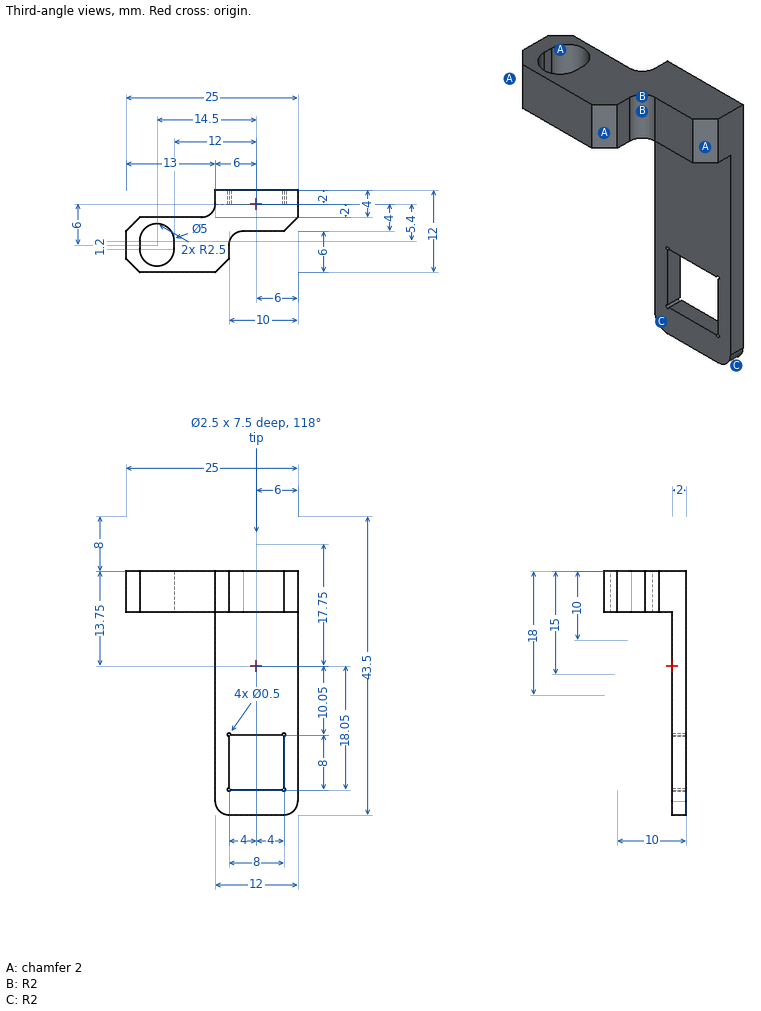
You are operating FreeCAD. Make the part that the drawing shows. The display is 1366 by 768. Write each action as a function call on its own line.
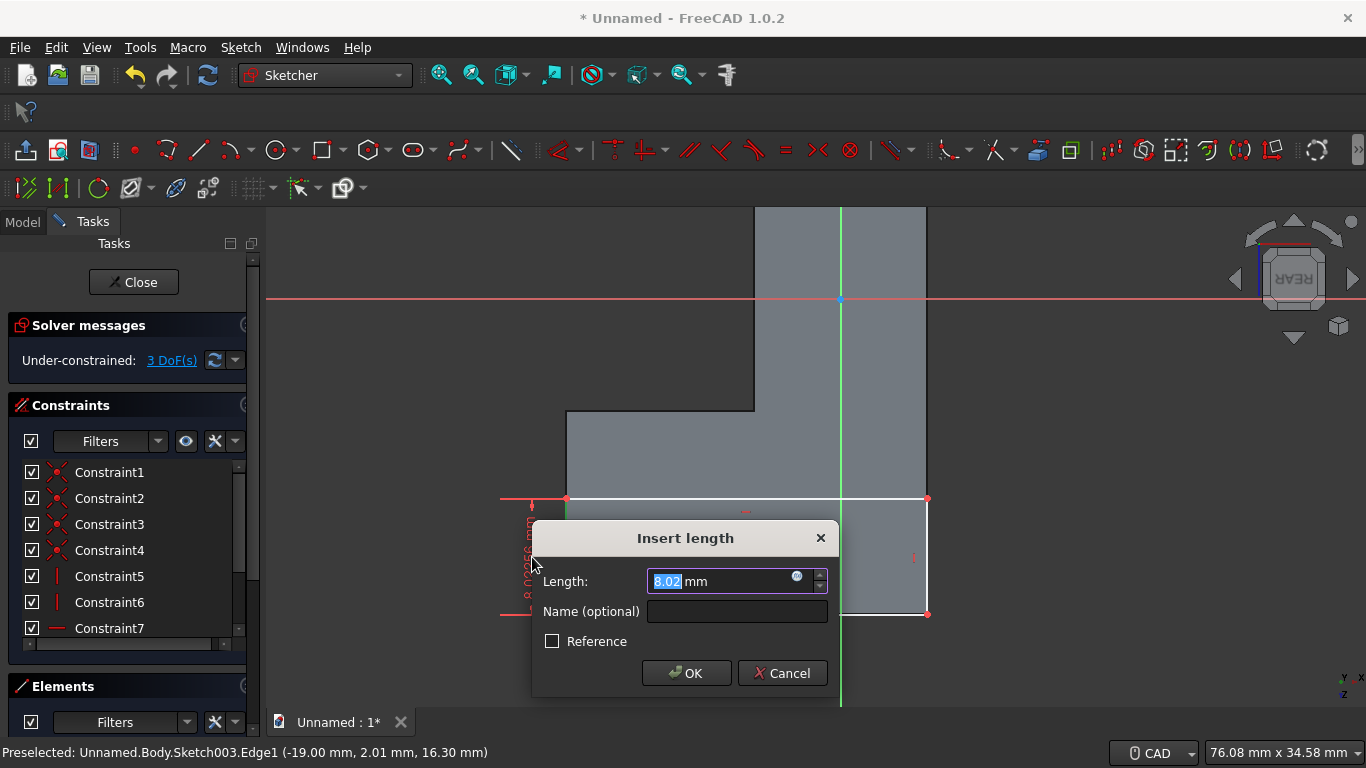
text(8)
key(Return)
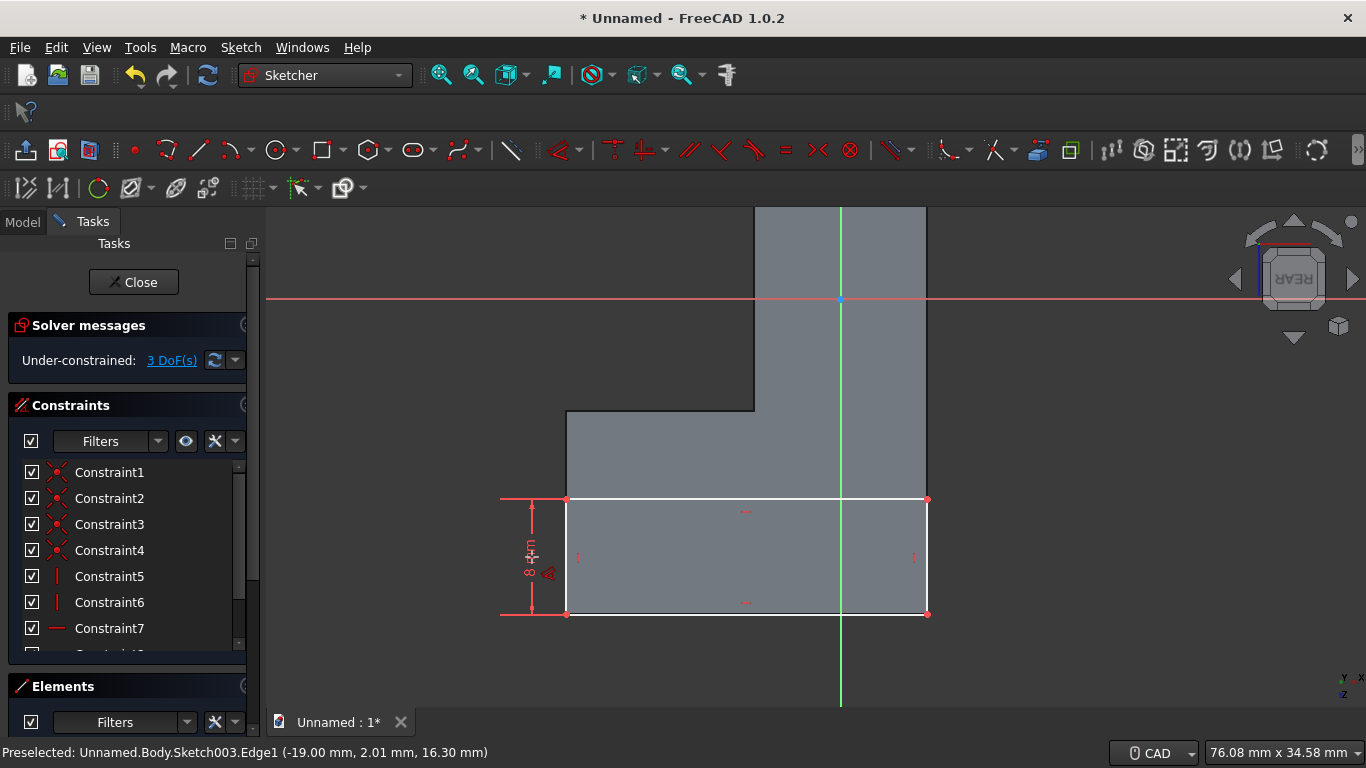
click(674, 615)
click(747, 649)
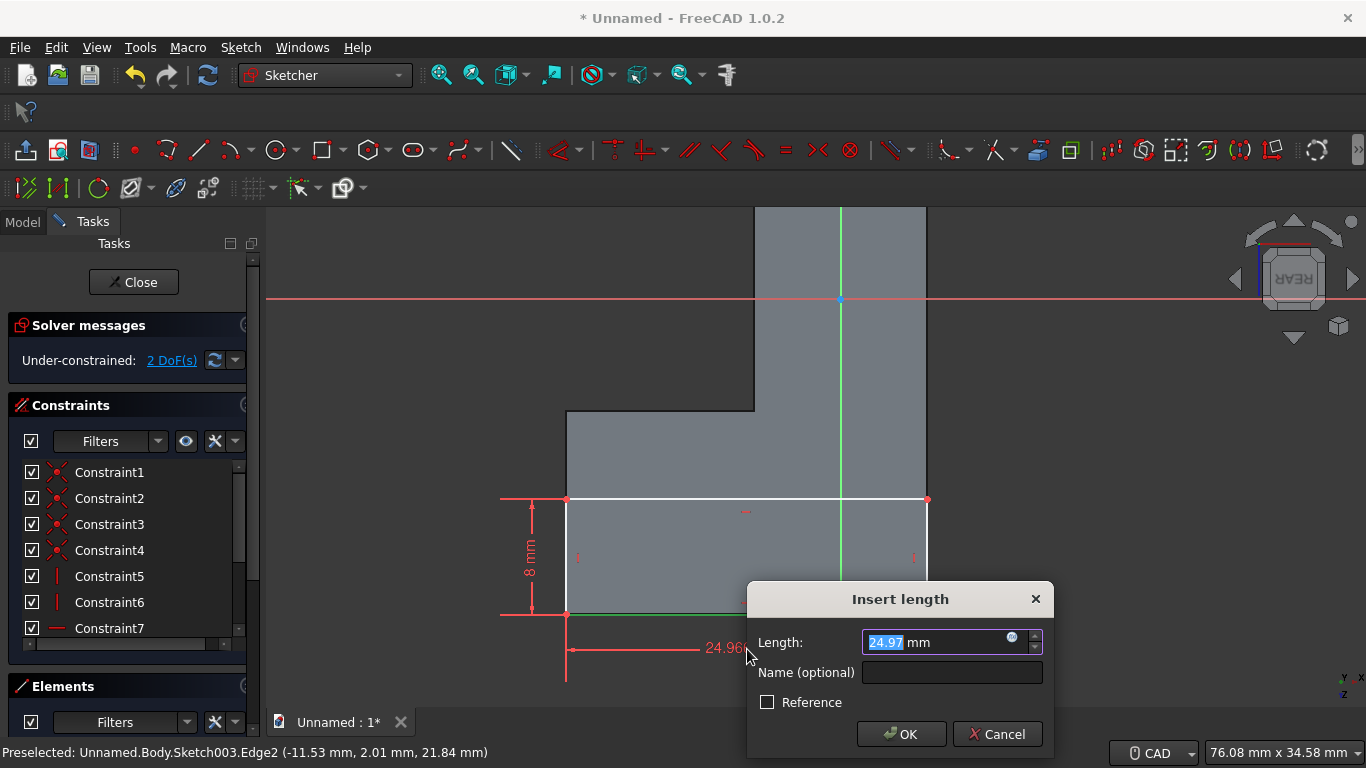
text(25)
key(Return)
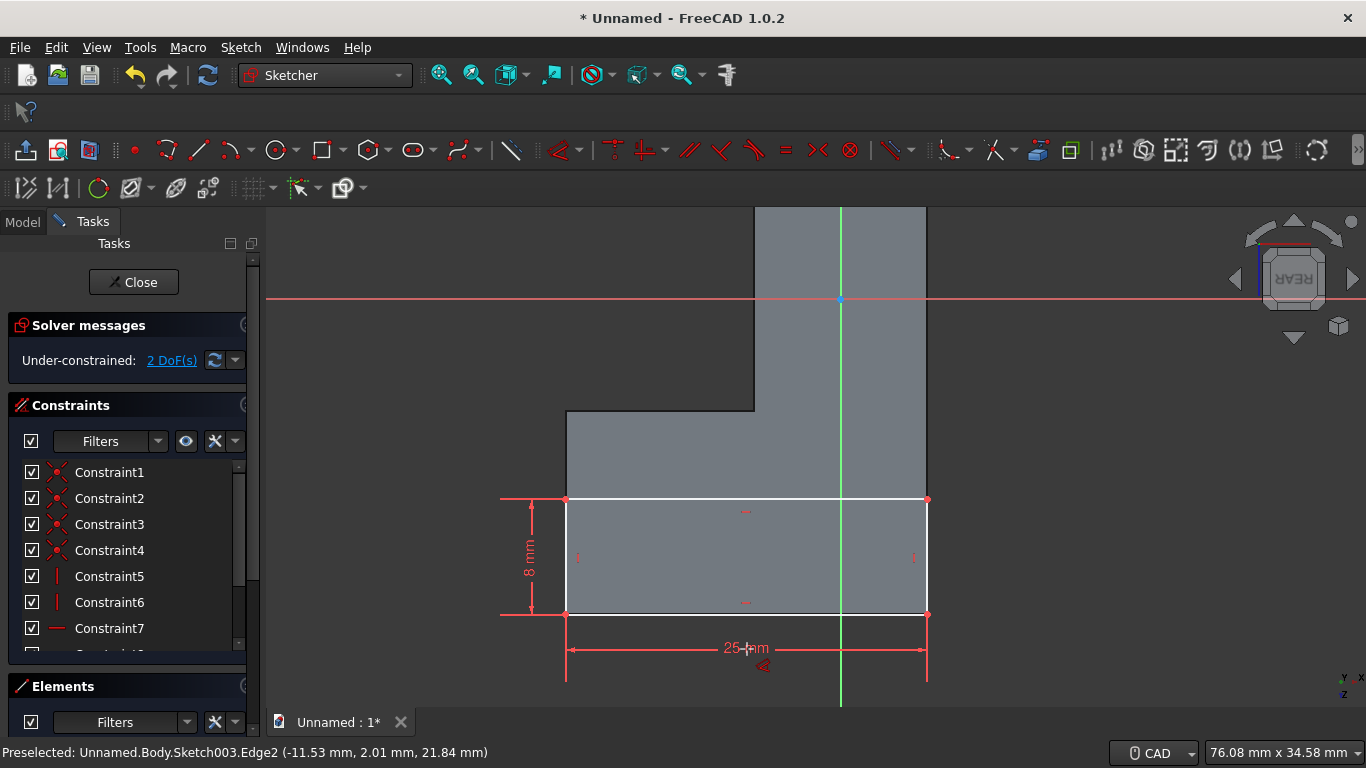
click(927, 615)
click(884, 649)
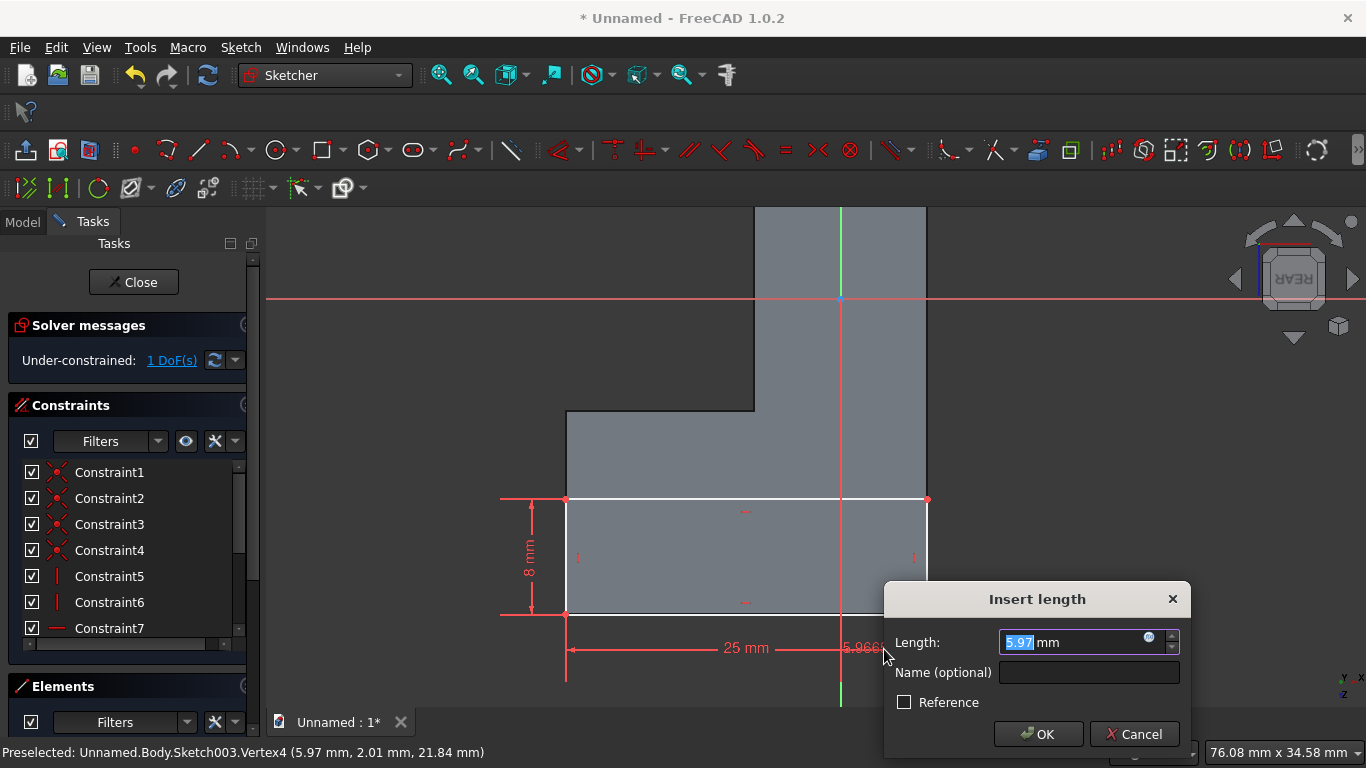
text(6)
key(Return)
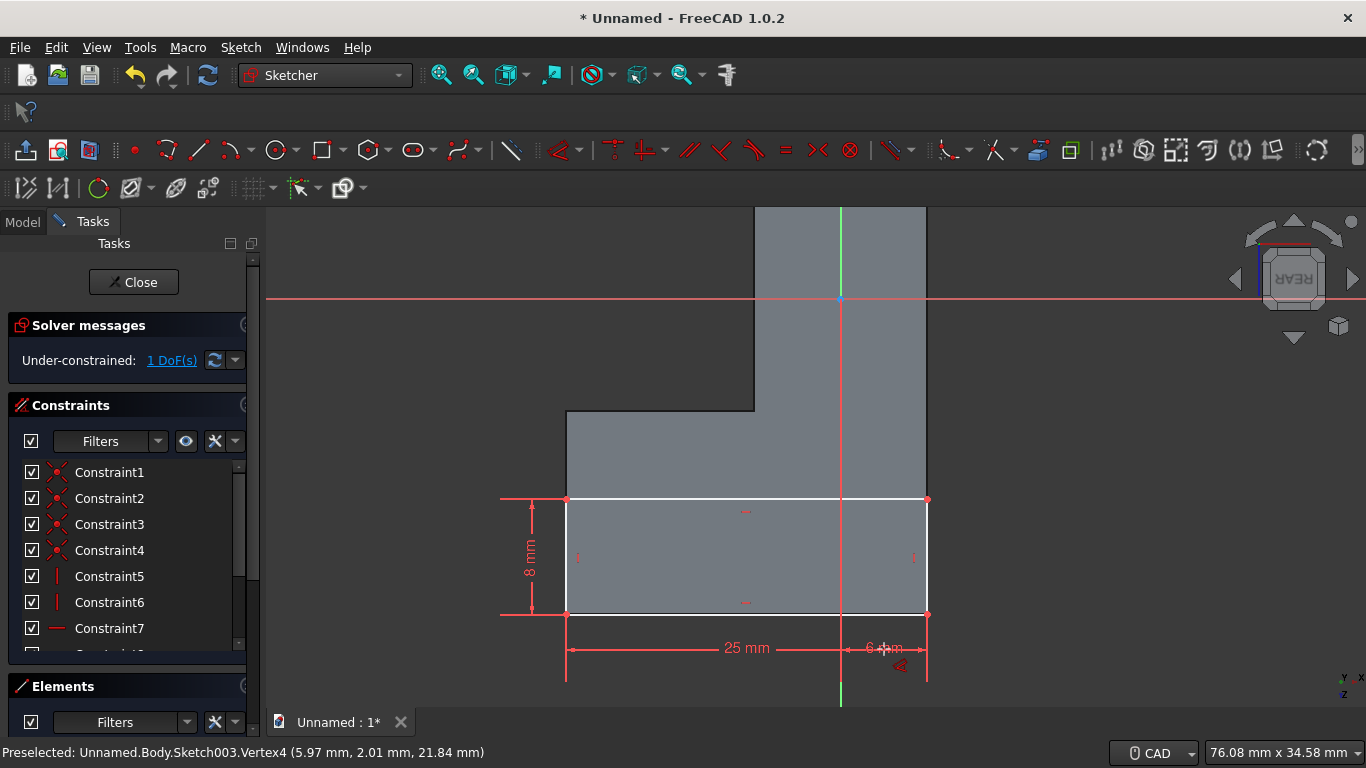
click(566, 499)
click(532, 399)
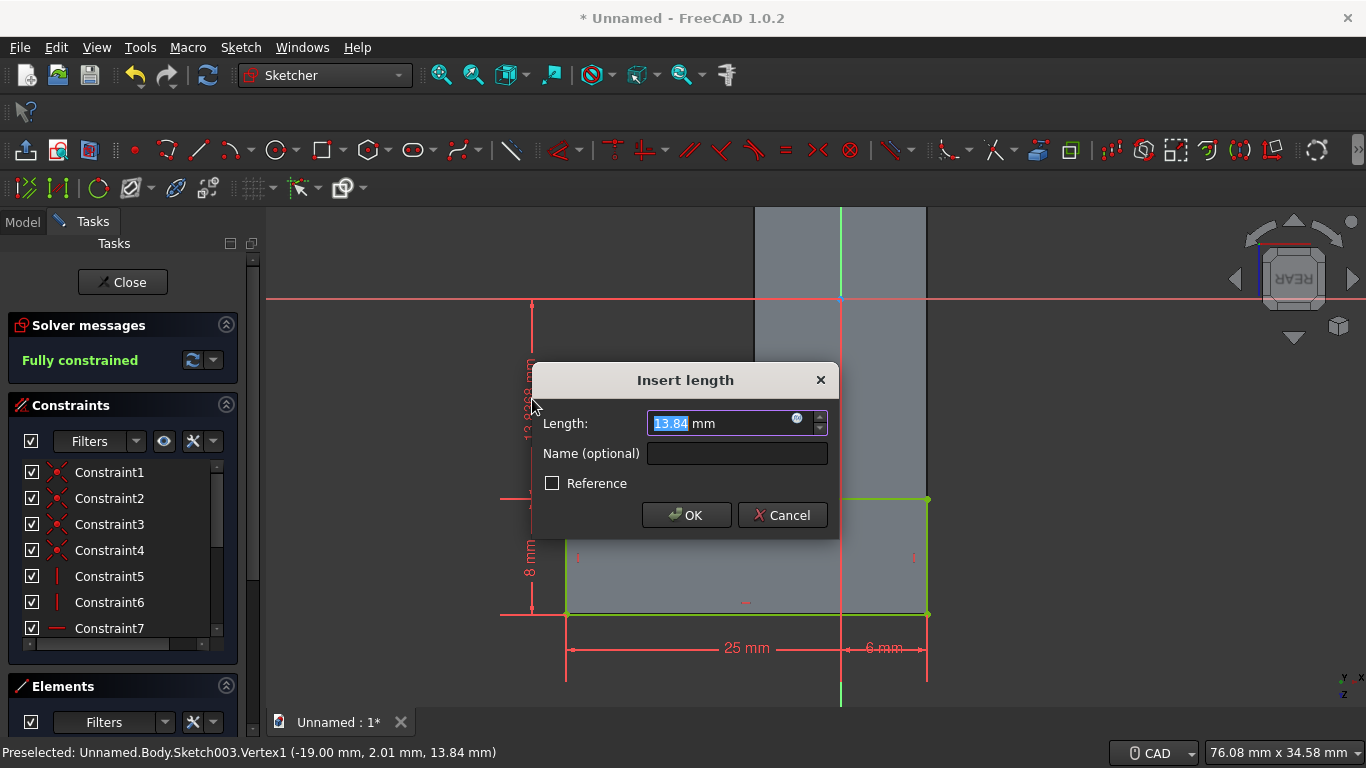
text(13.75)
key(Return)
key(Escape)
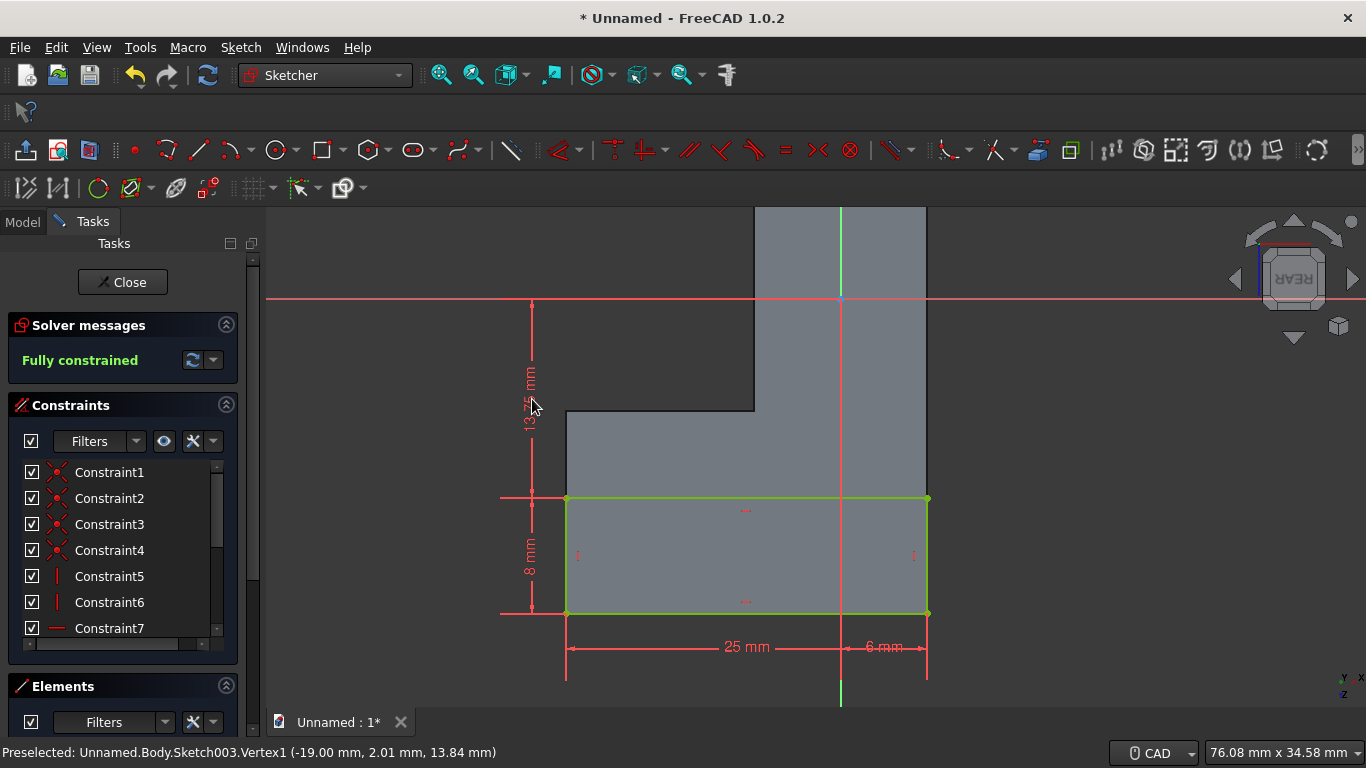
click(123, 282)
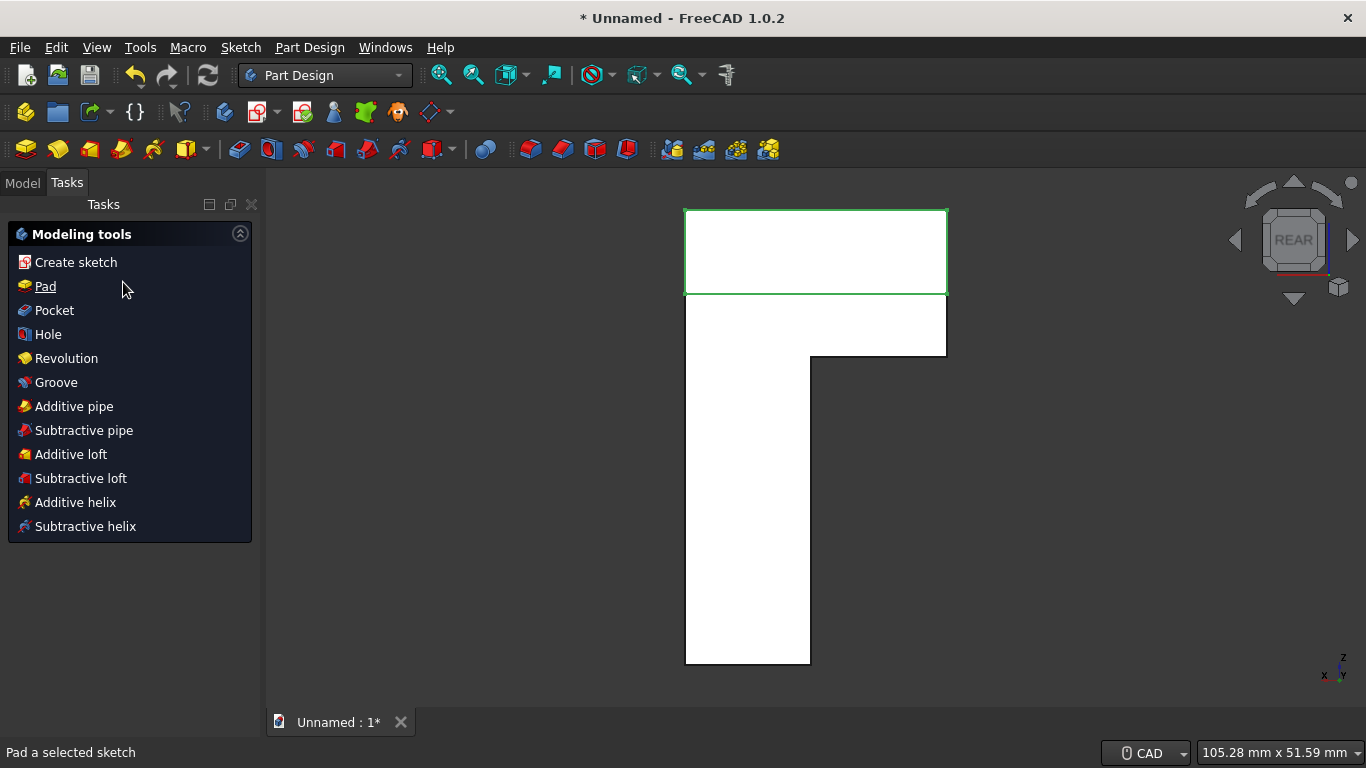
click(240, 150)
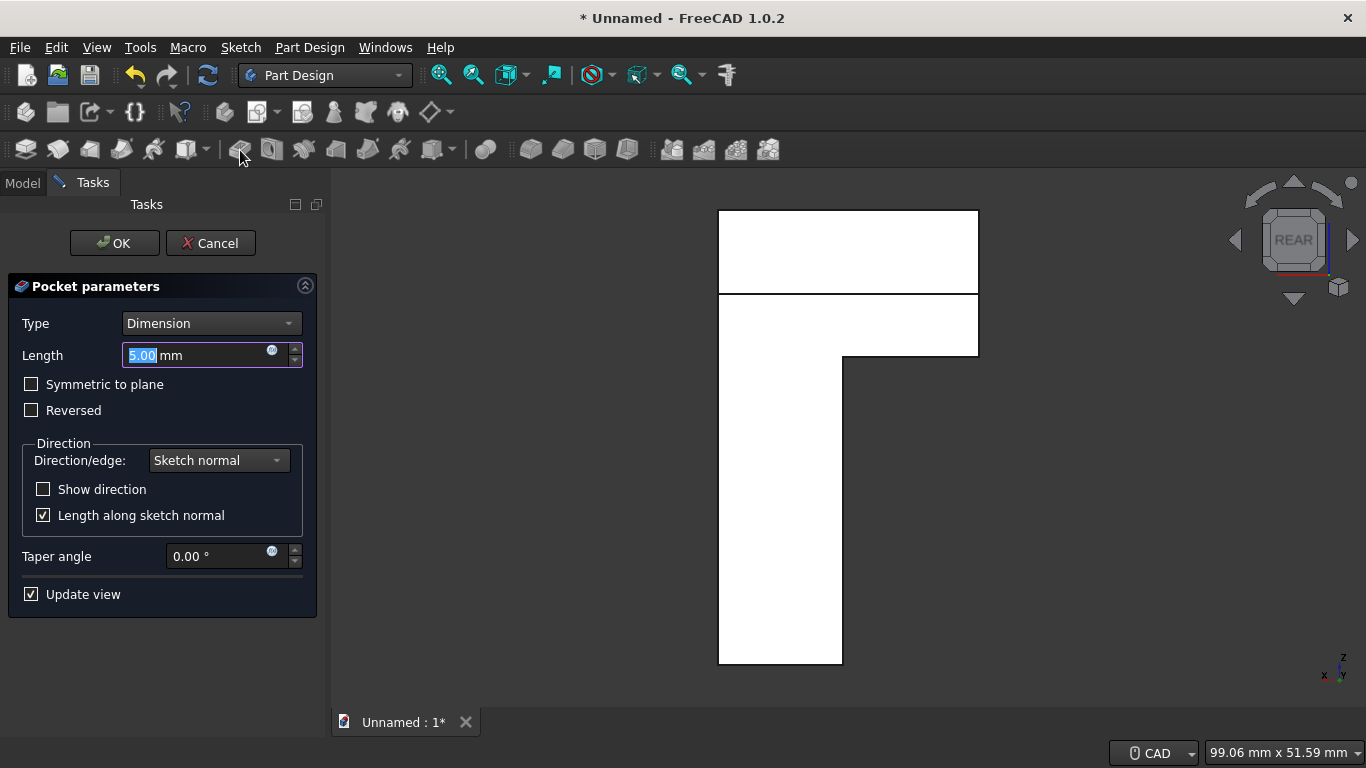
click(212, 324)